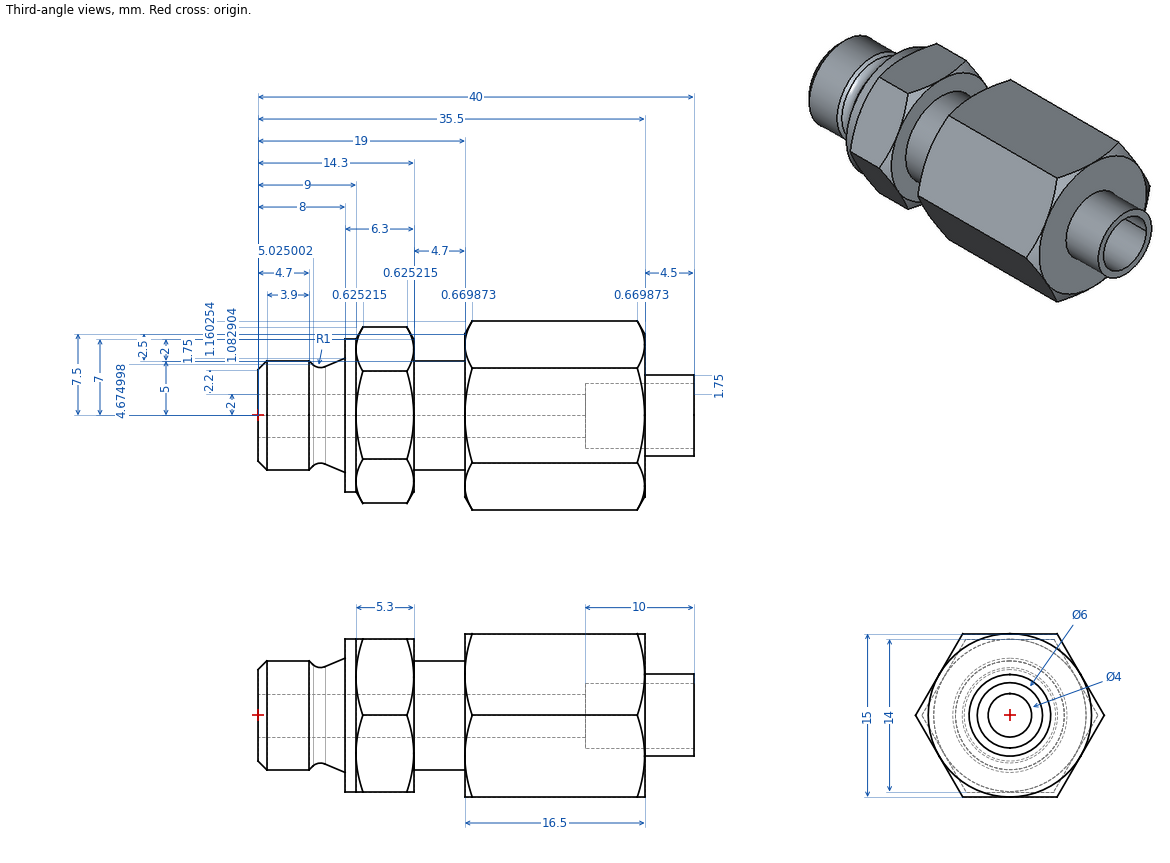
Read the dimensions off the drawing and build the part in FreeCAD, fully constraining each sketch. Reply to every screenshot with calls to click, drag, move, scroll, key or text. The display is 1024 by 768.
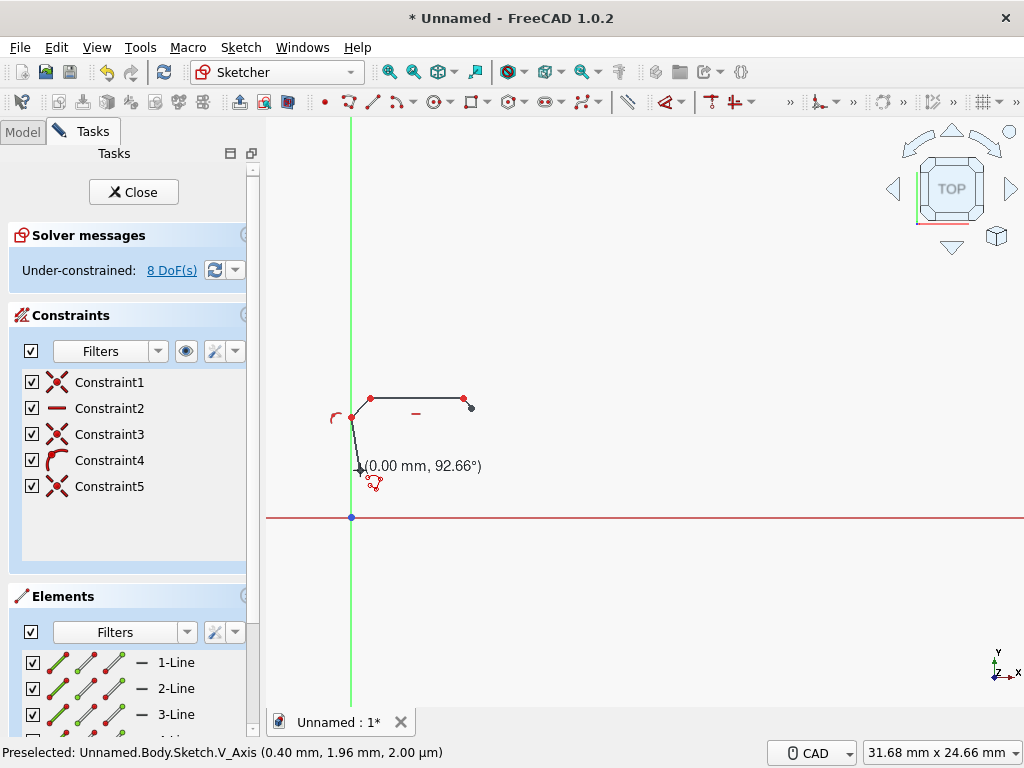
scroll(370, 399, down, 4)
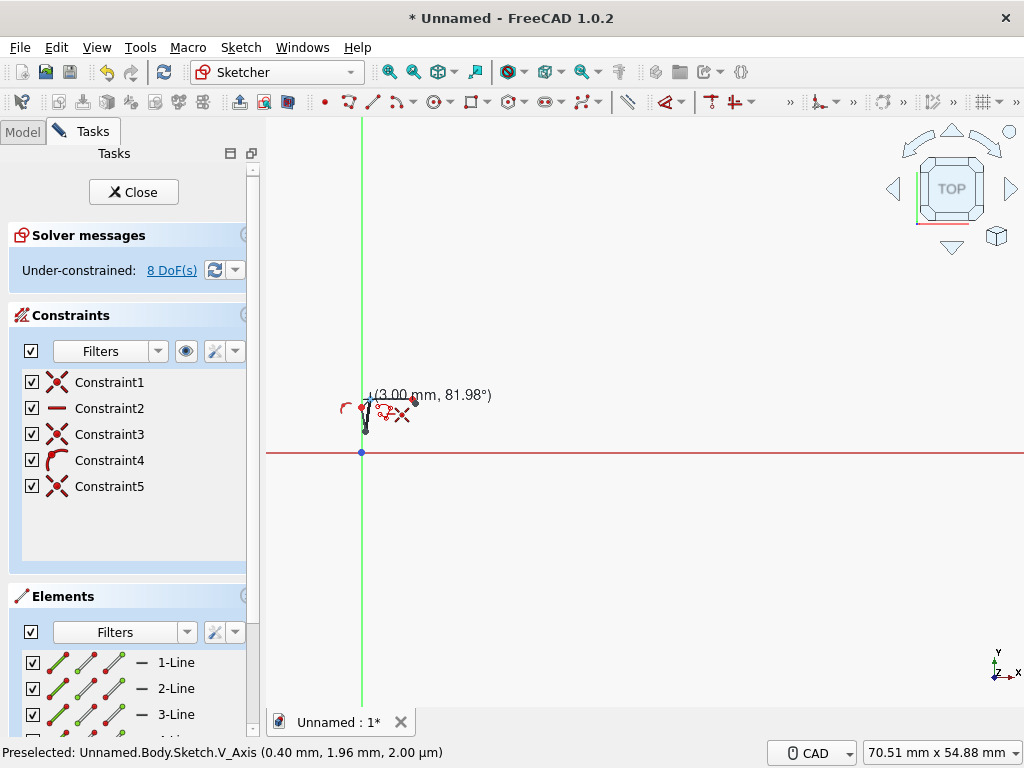
click(792, 431)
click(792, 412)
click(743, 412)
click(743, 372)
click(566, 372)
click(566, 399)
click(515, 399)
click(515, 377)
click(448, 377)
click(448, 396)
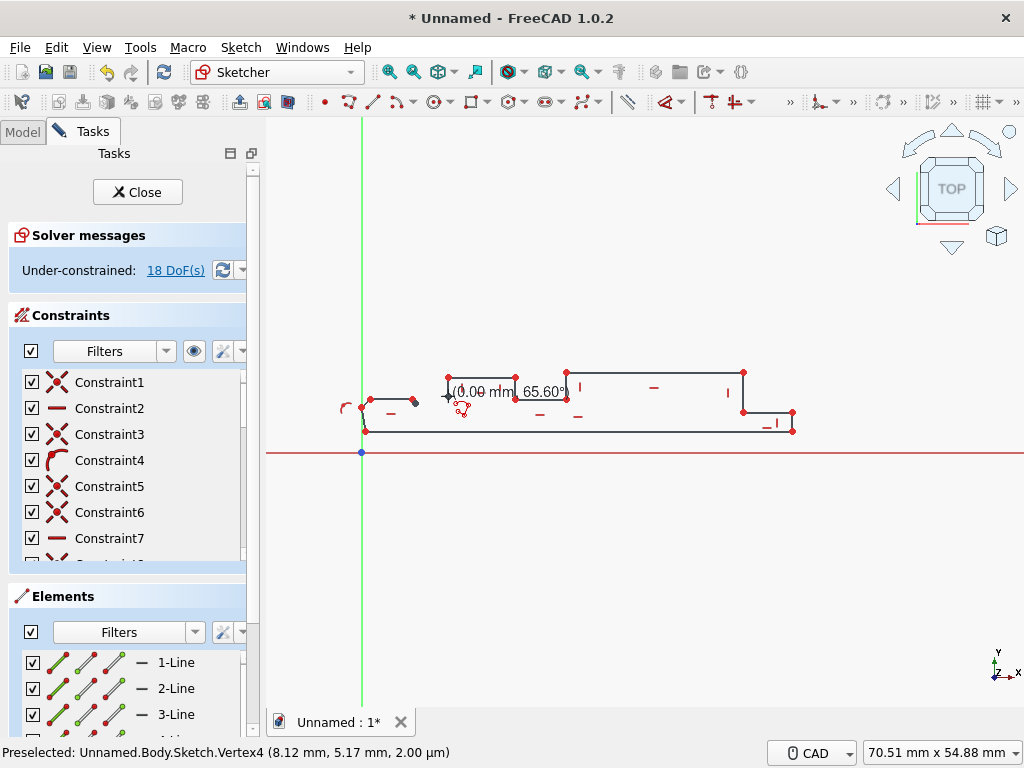
scroll(427, 405, up, 2)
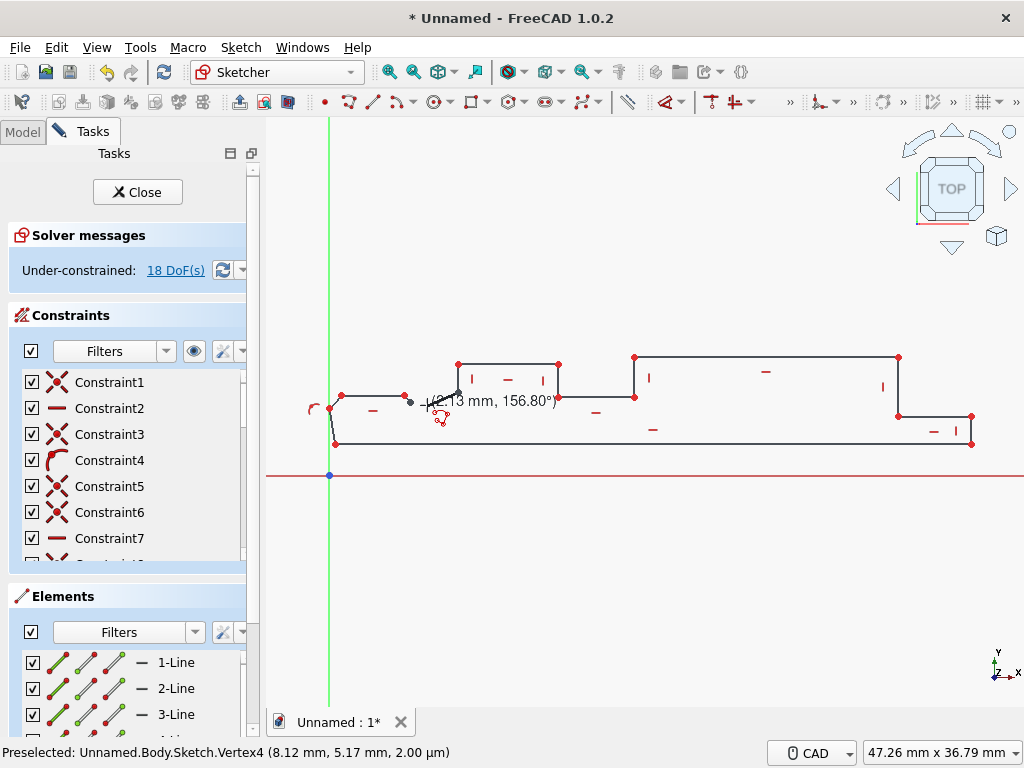
click(428, 404)
right_click(428, 404)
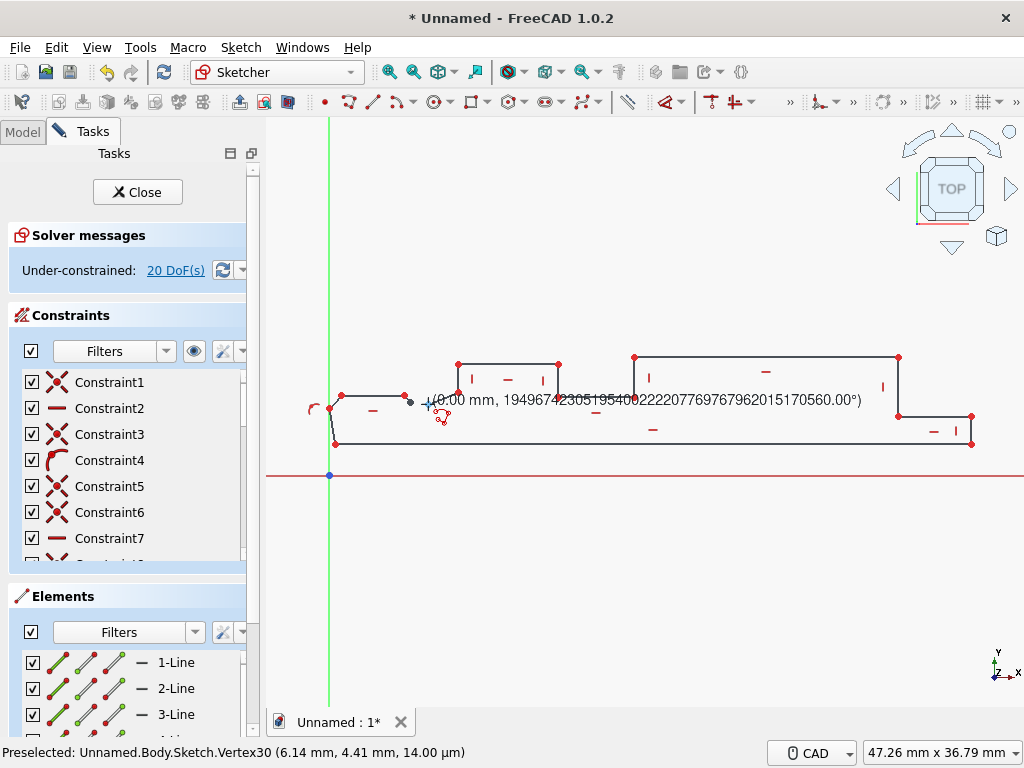
key(g)
key(3)
key(a)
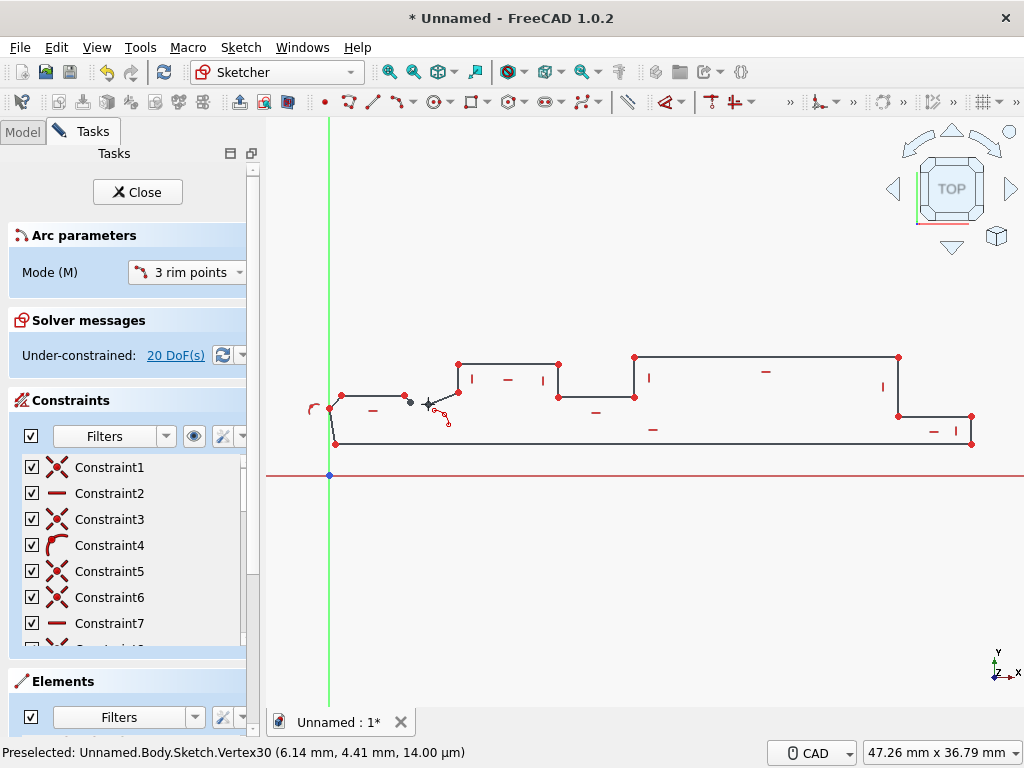
click(428, 405)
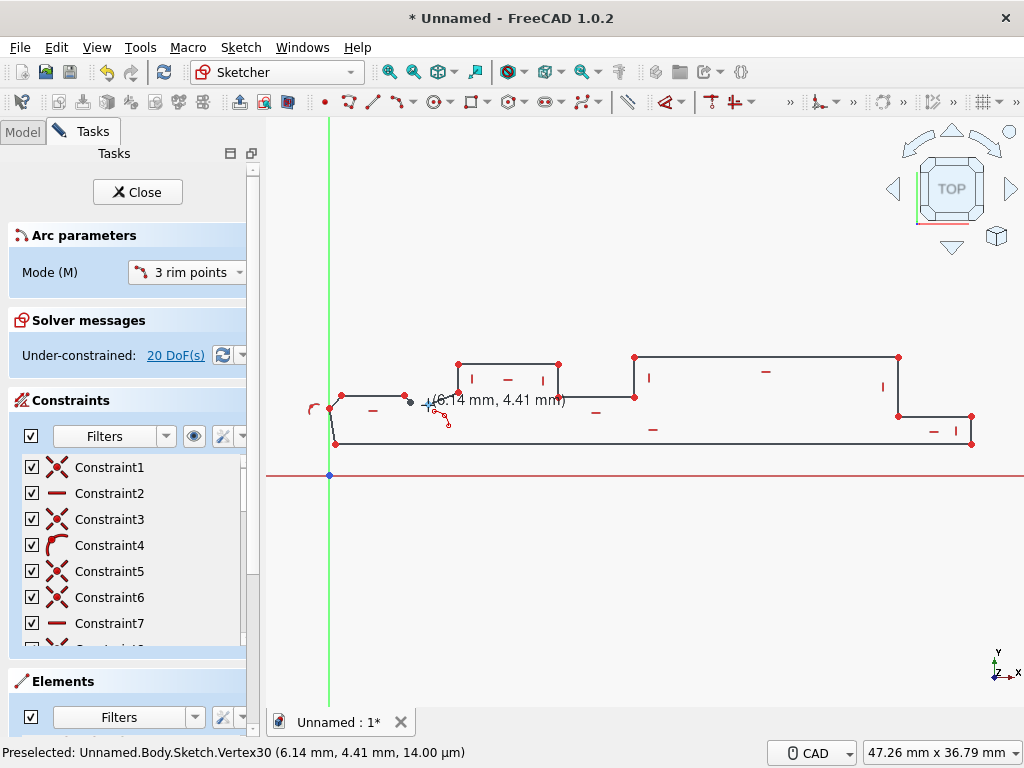
scroll(410, 401, up, 8)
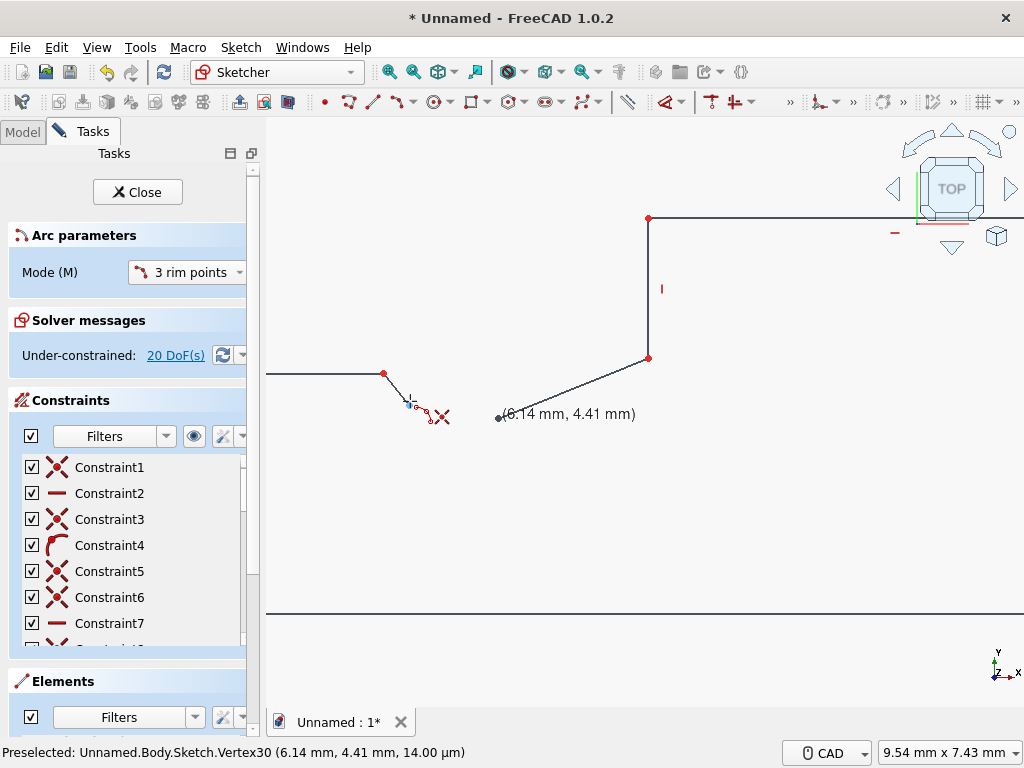
click(409, 406)
click(450, 420)
key(Escape)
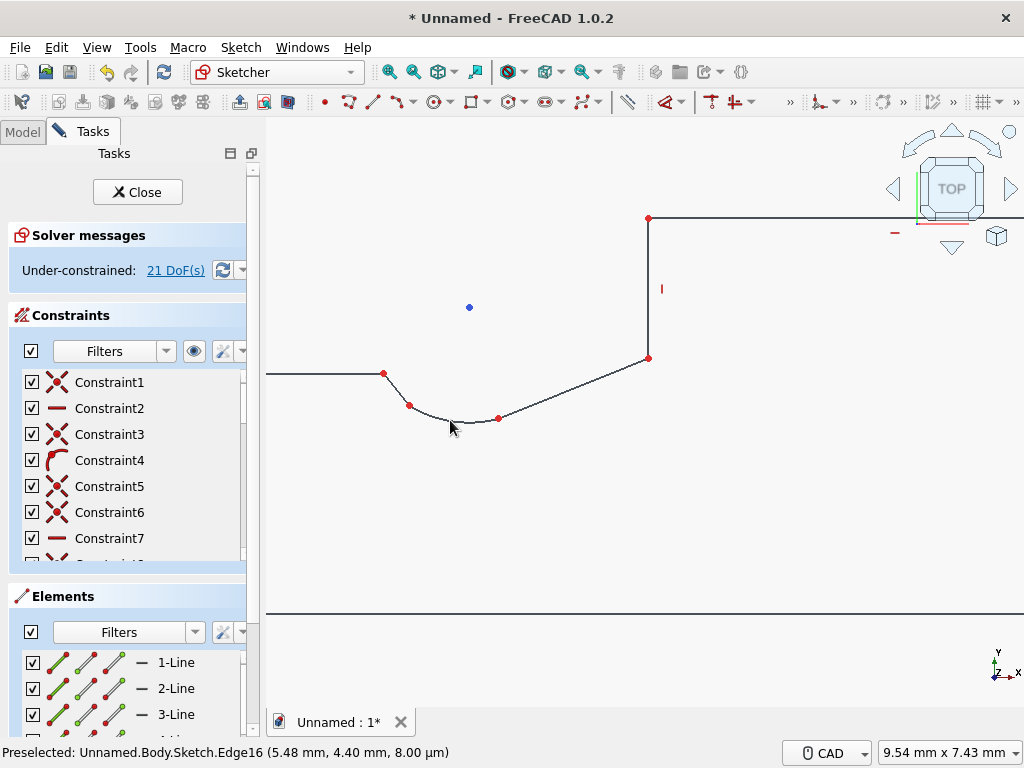
click(402, 396)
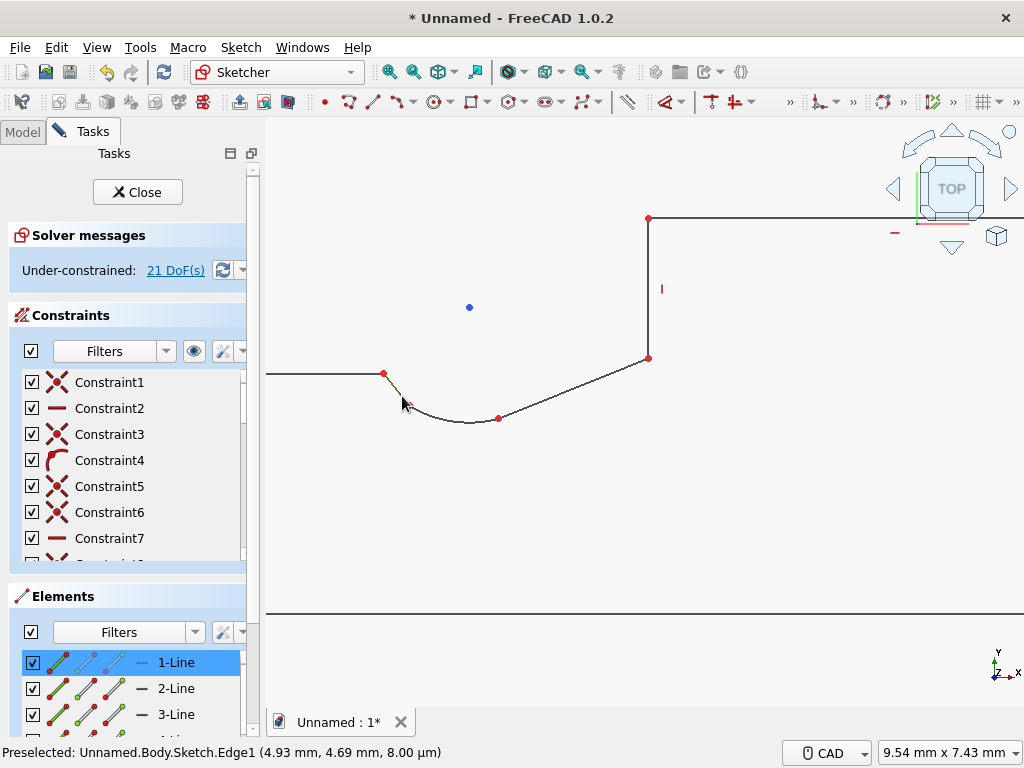
click(435, 417)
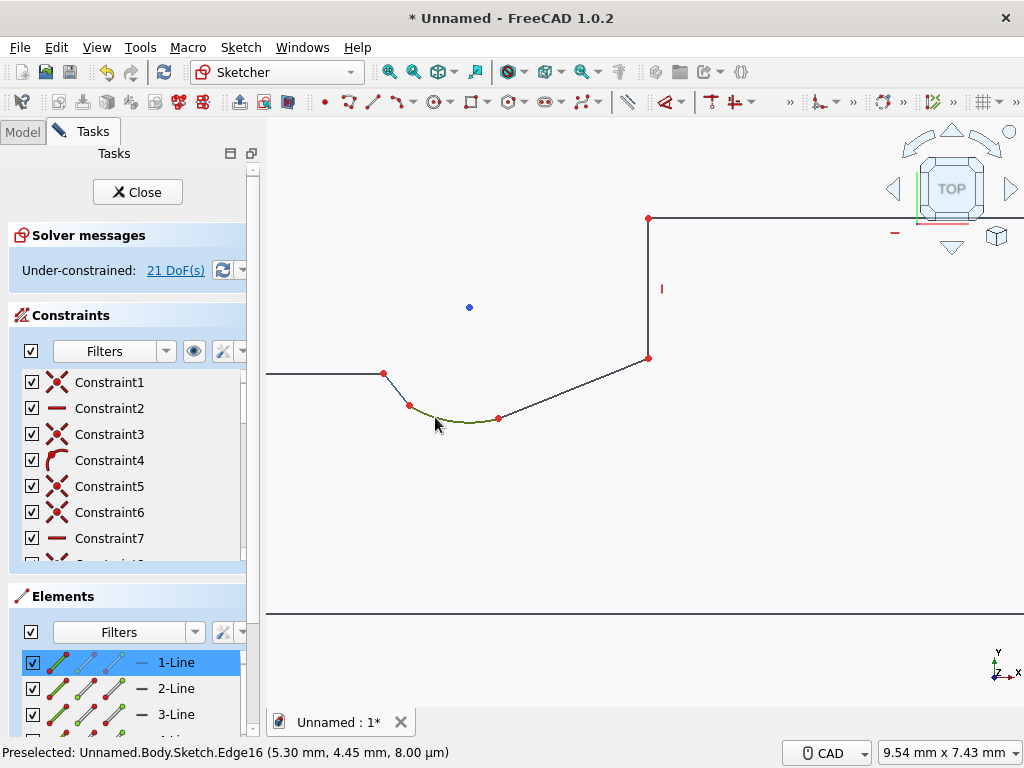
key(t)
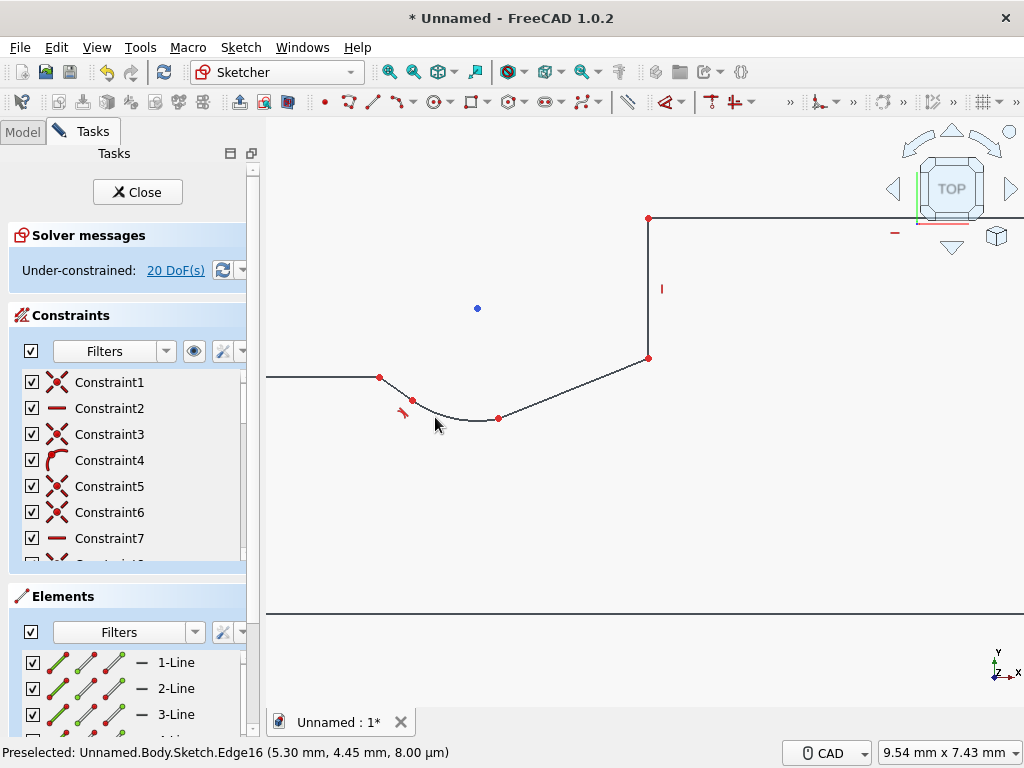
scroll(416, 403, down, 10)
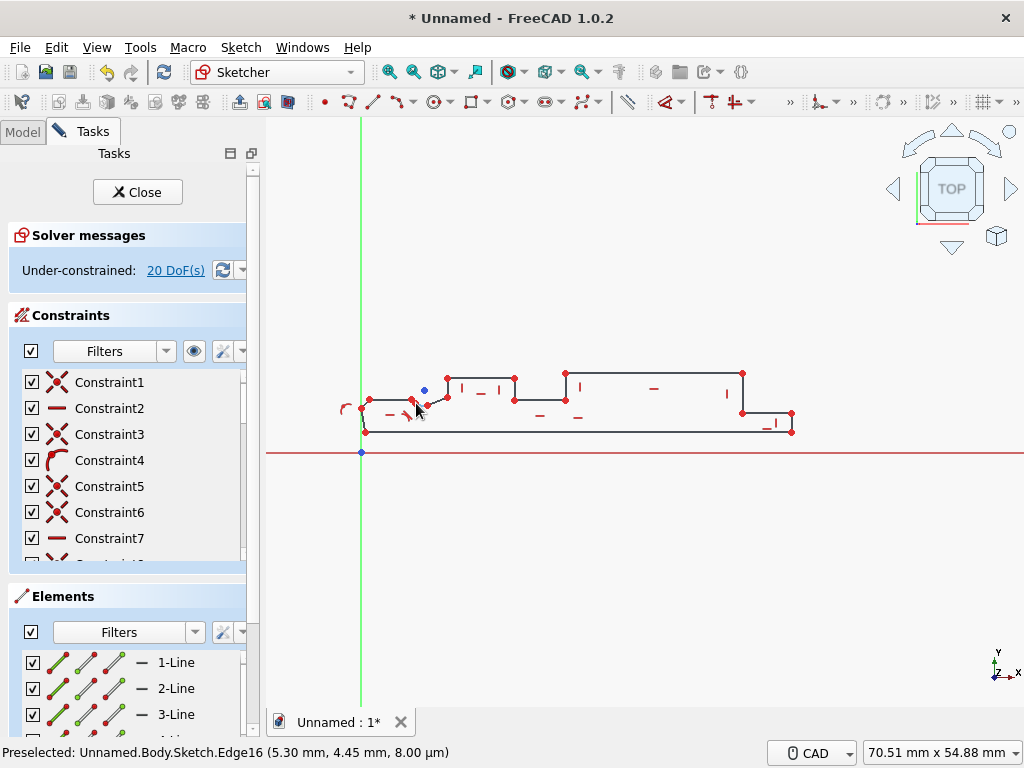
scroll(442, 400, up, 4)